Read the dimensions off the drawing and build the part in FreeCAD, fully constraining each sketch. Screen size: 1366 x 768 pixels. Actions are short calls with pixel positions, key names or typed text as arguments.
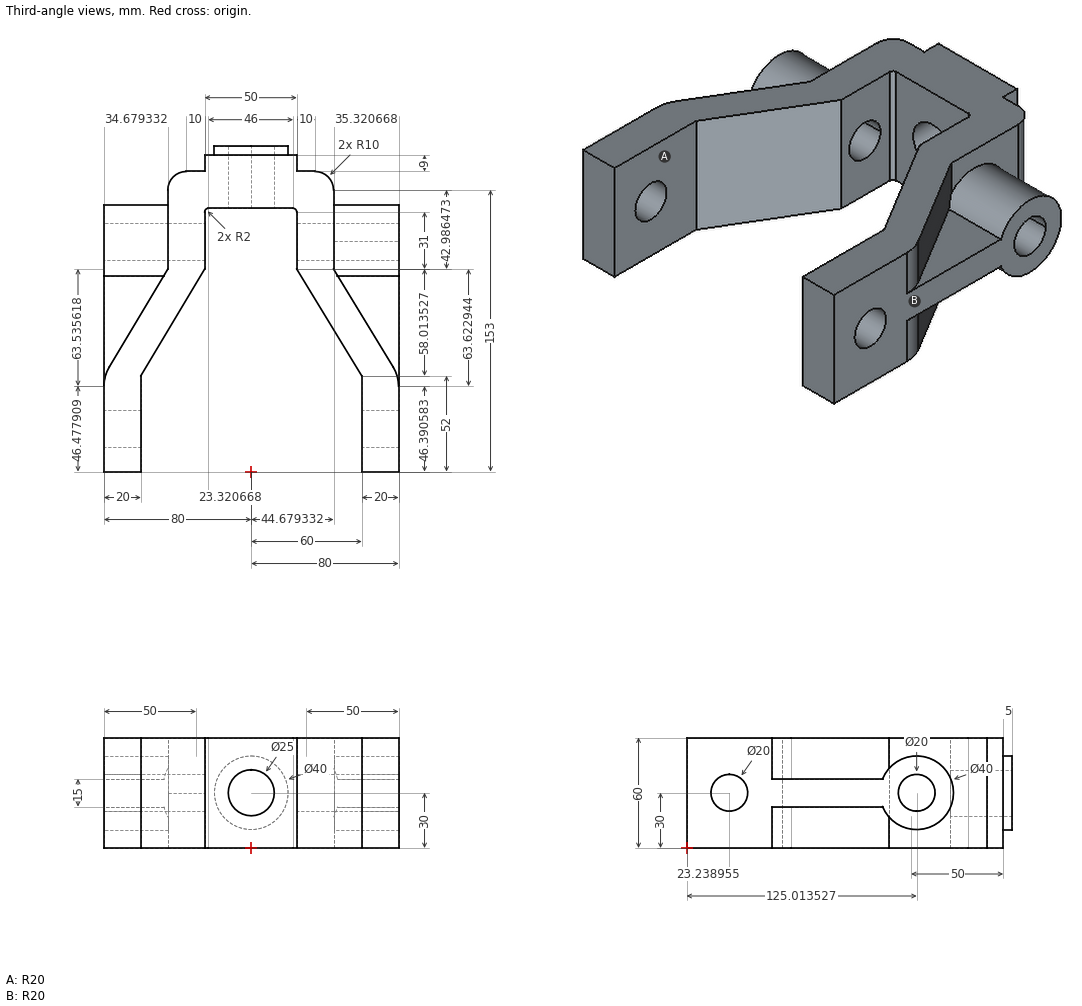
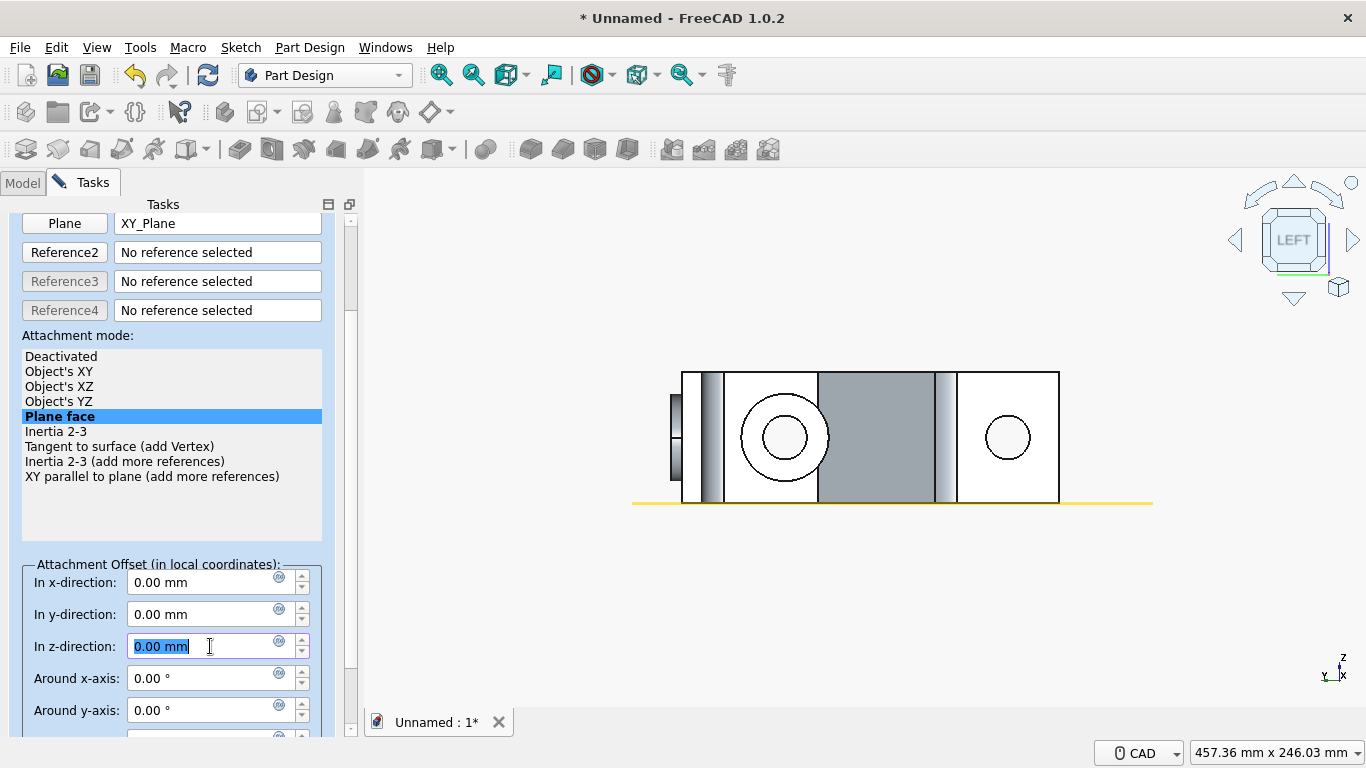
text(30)
key(Tab)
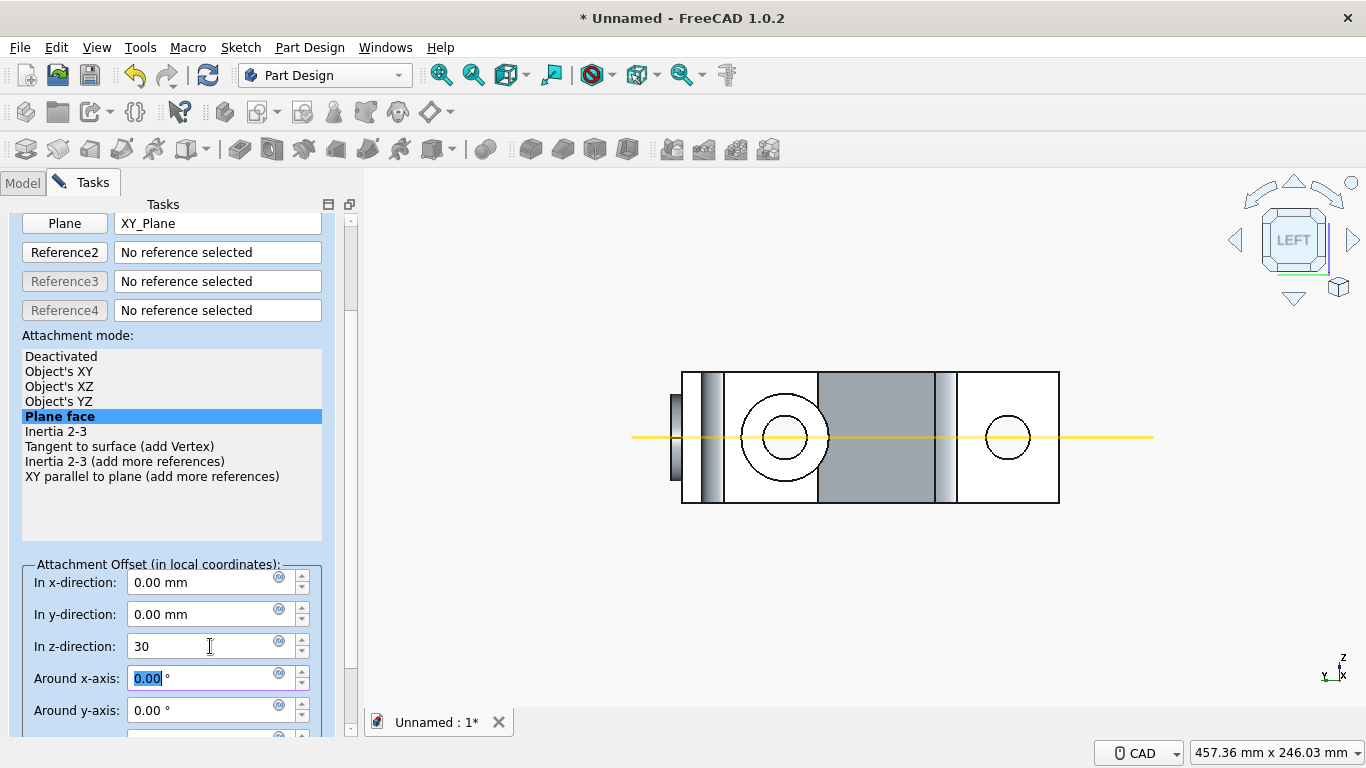
scroll(351, 475, up, 3)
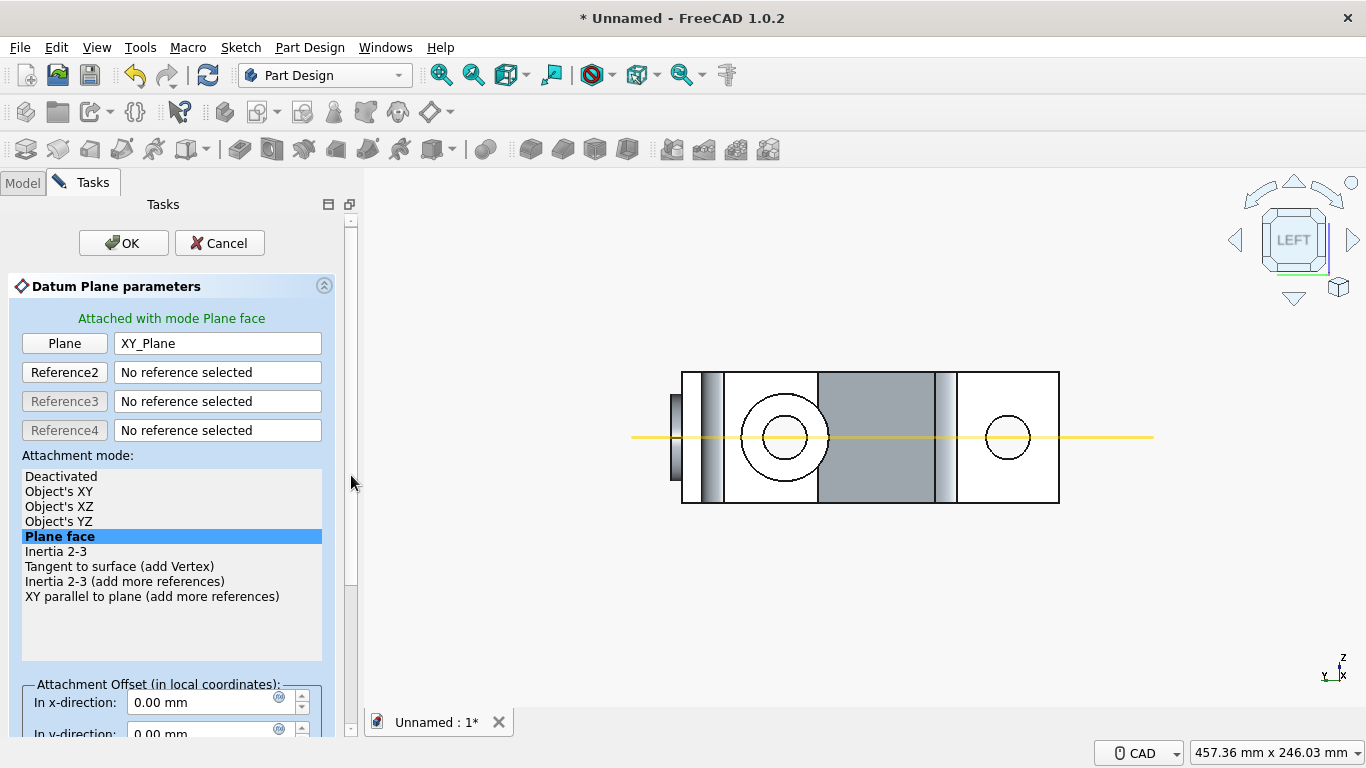
click(124, 243)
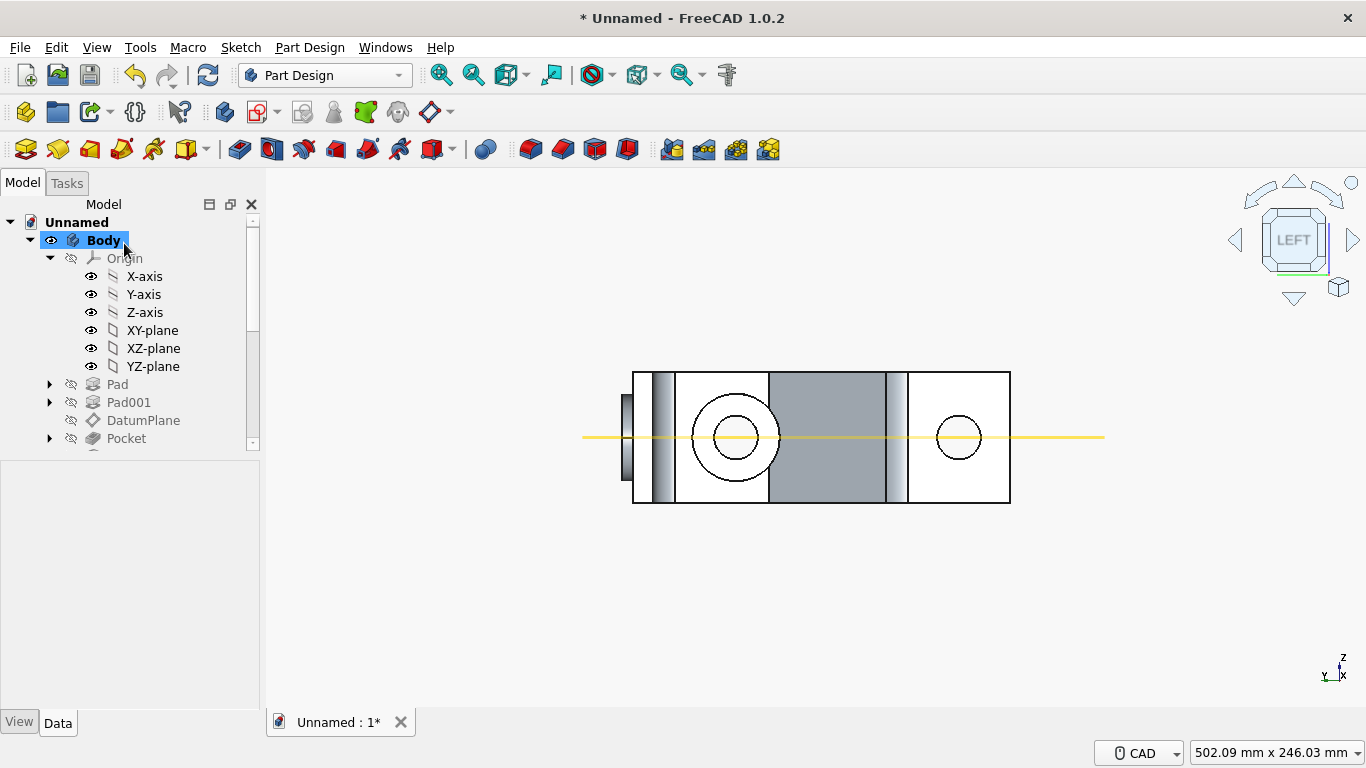
scroll(100, 326, down, 3)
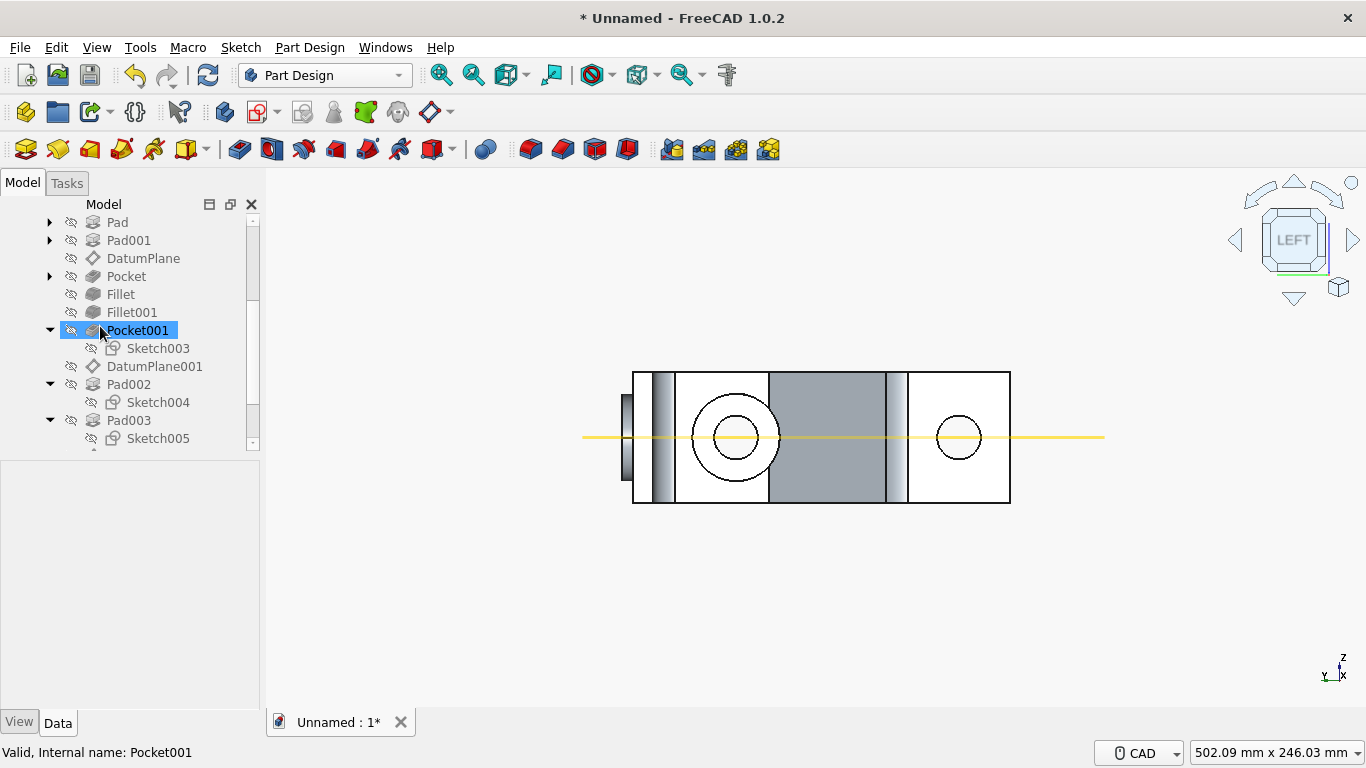
scroll(140, 326, up, 15)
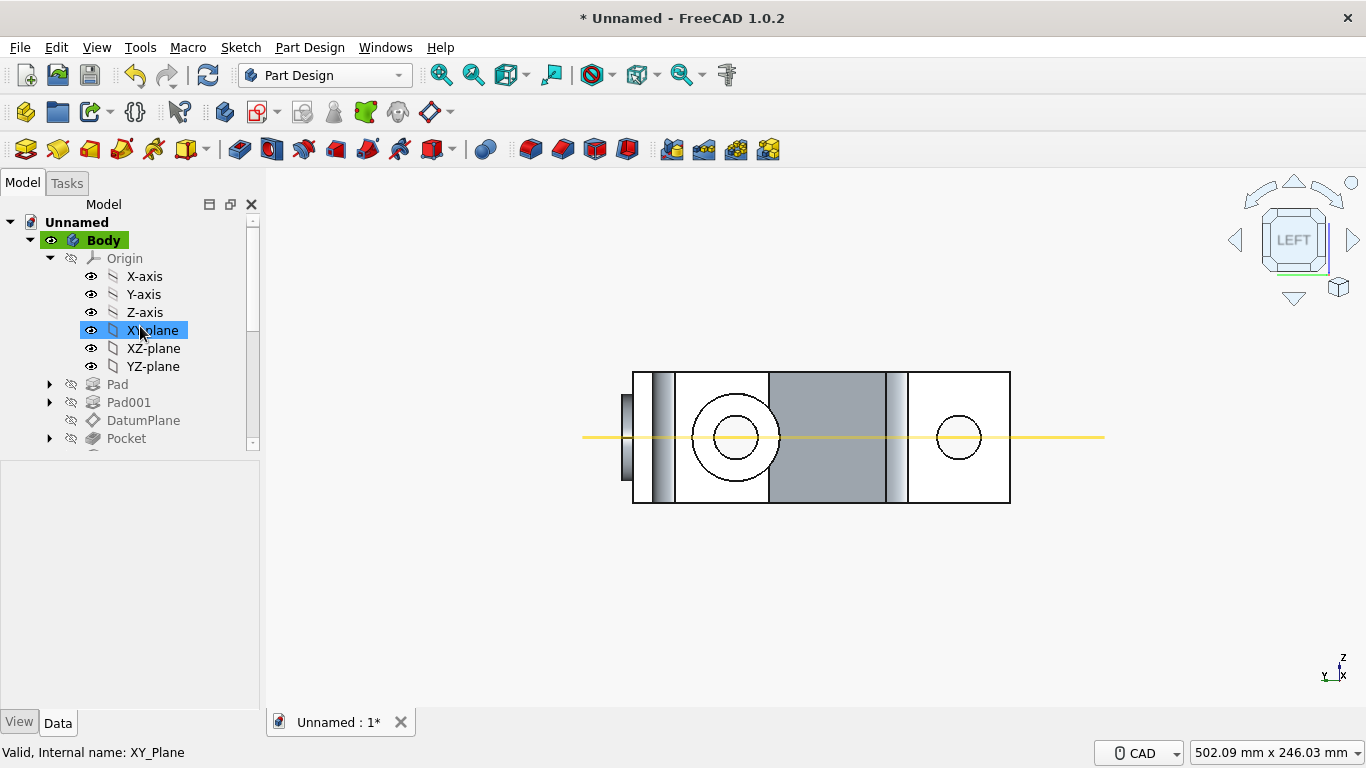
scroll(100, 326, down, 6)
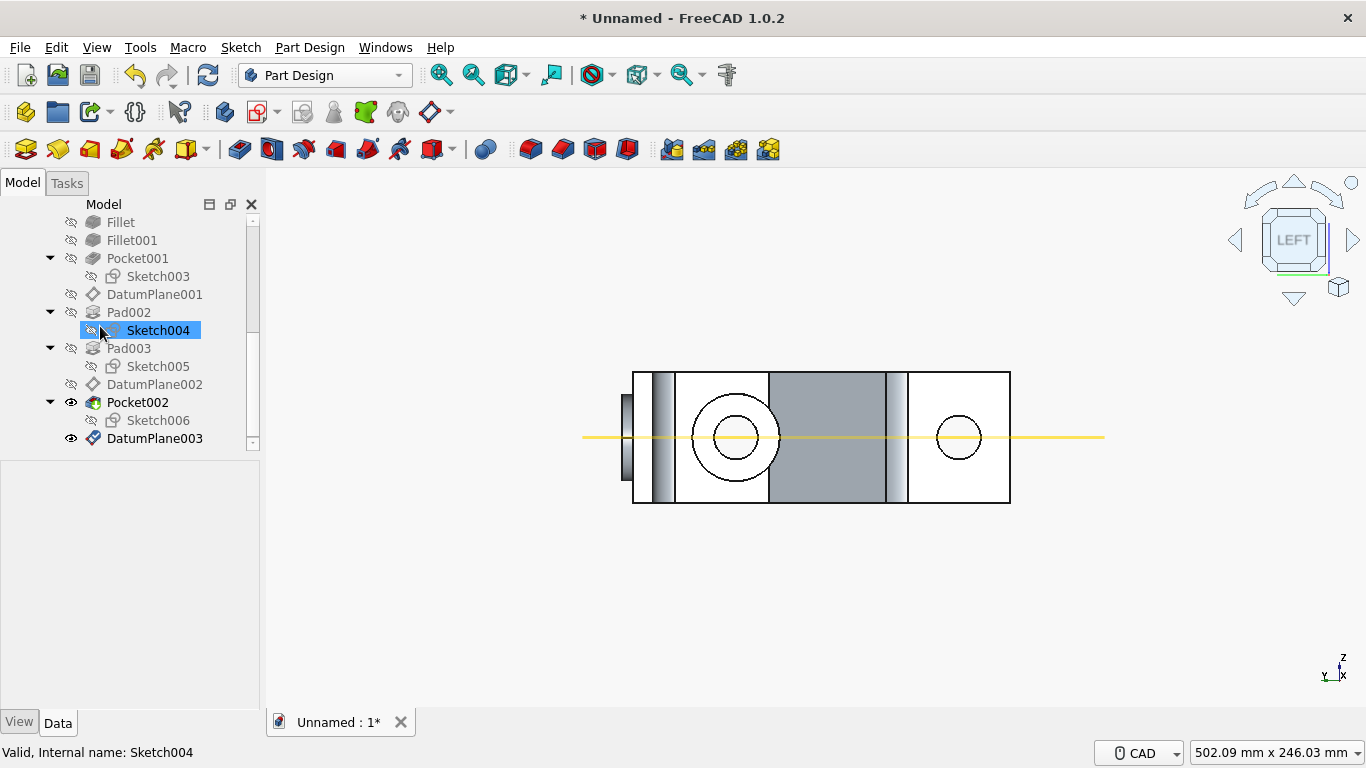
click(116, 438)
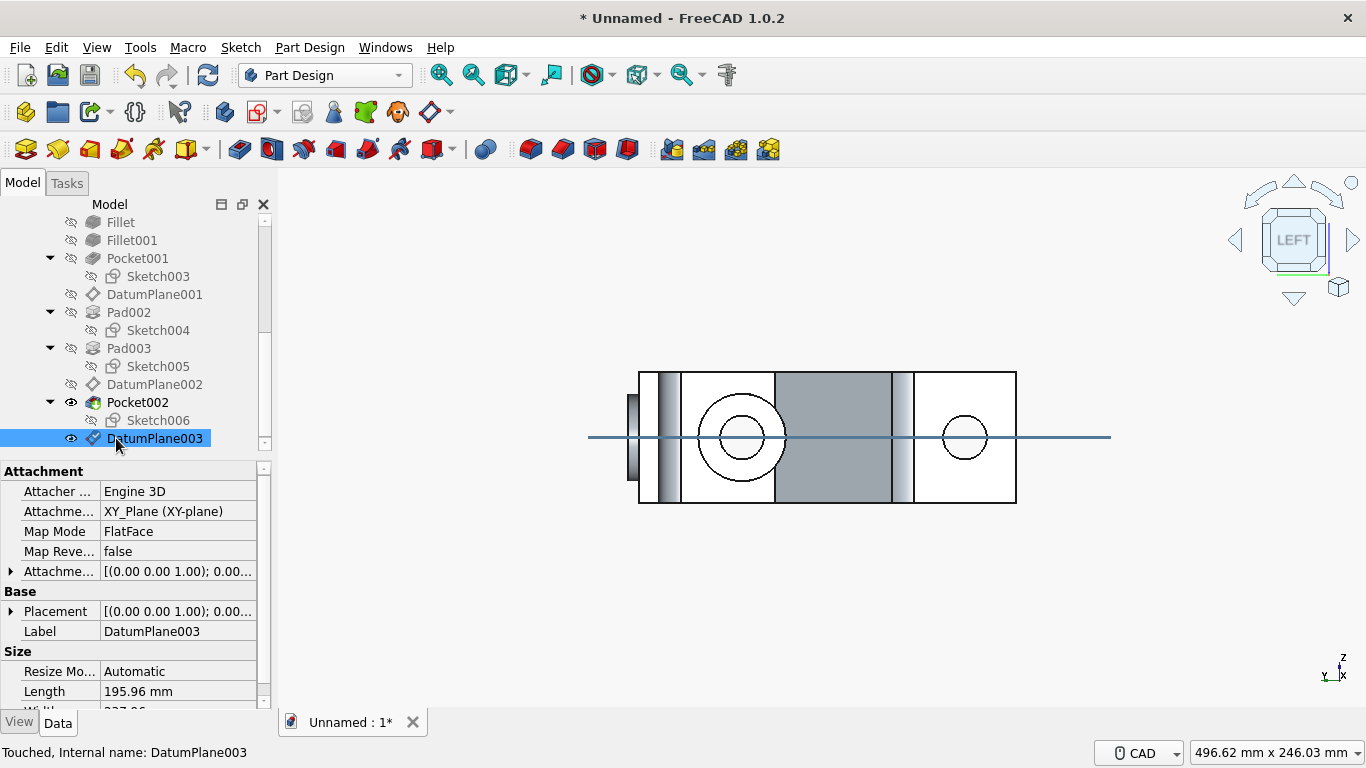
click(258, 112)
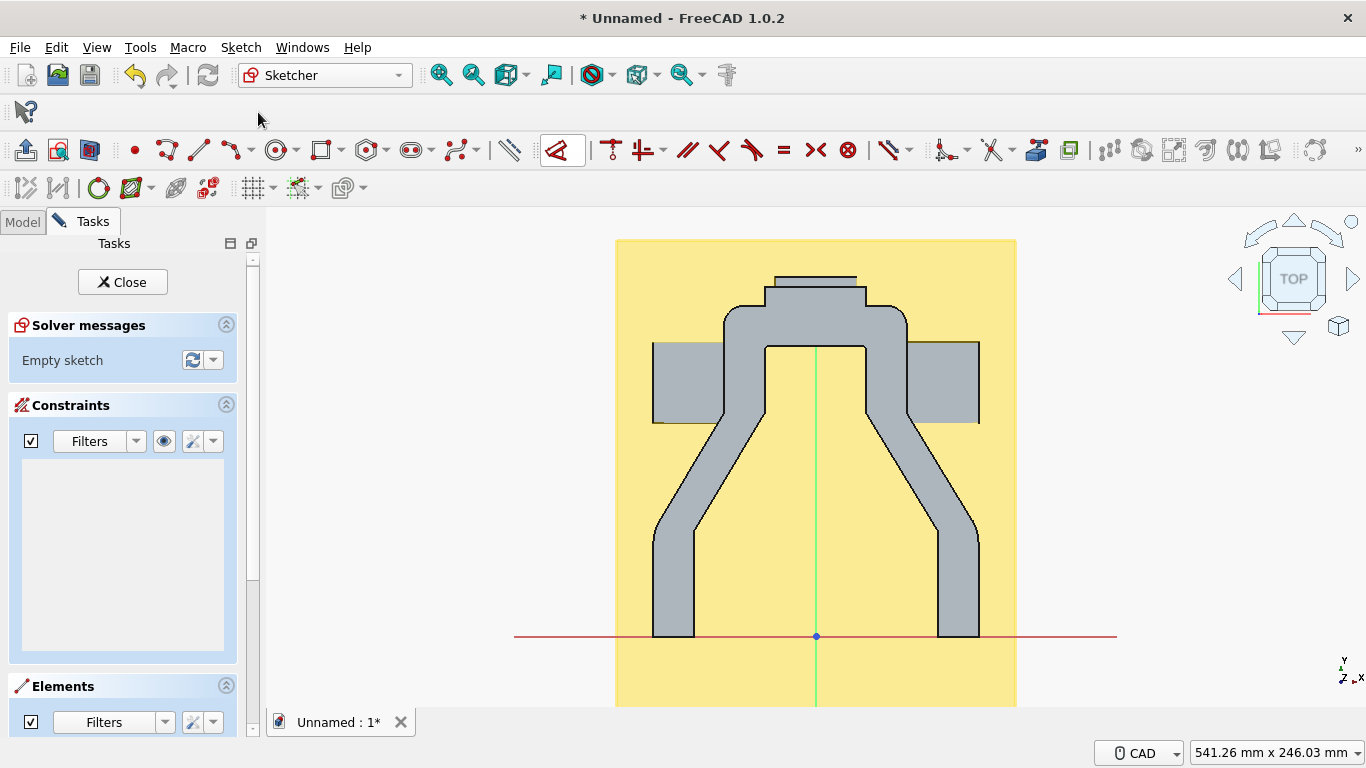
key(q)
key(s)